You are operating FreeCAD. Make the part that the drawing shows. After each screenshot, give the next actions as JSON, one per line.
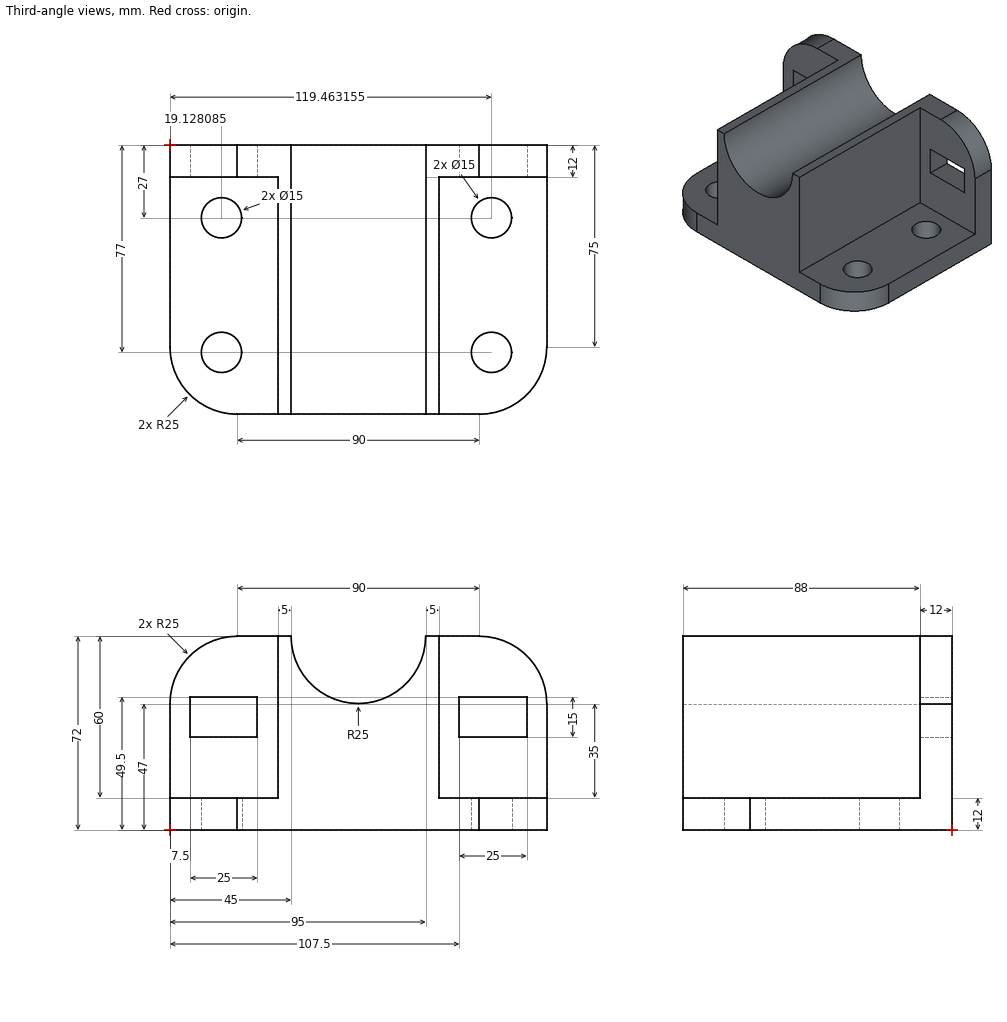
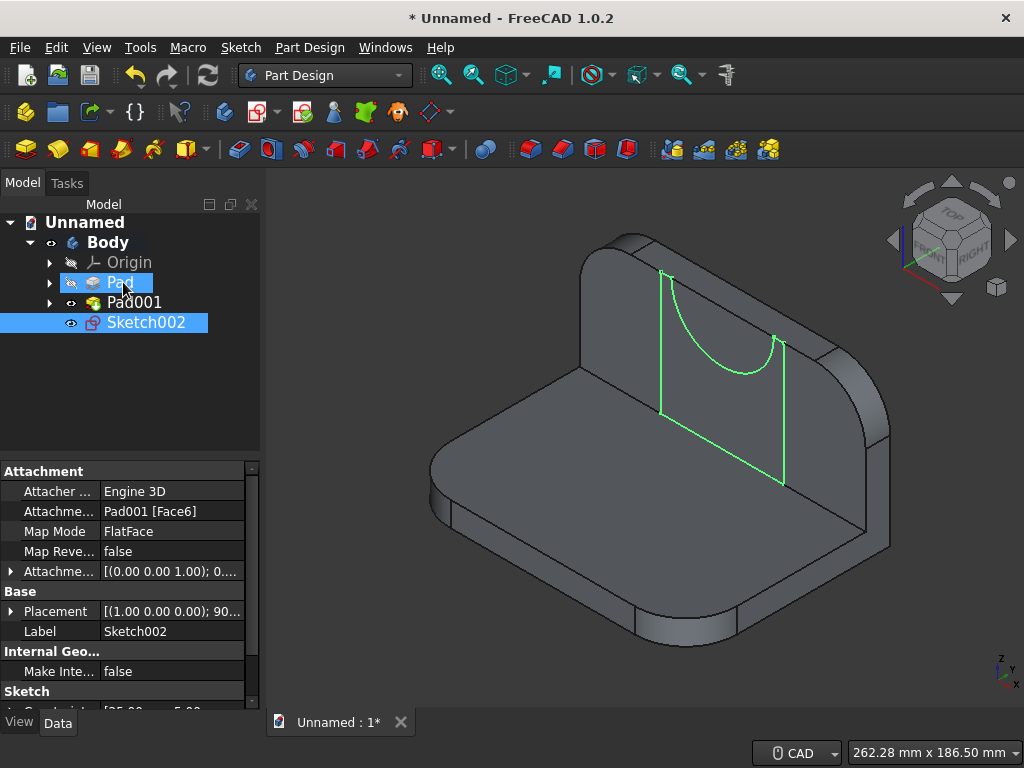
{"action": "left_click", "coordinate": [26, 150]}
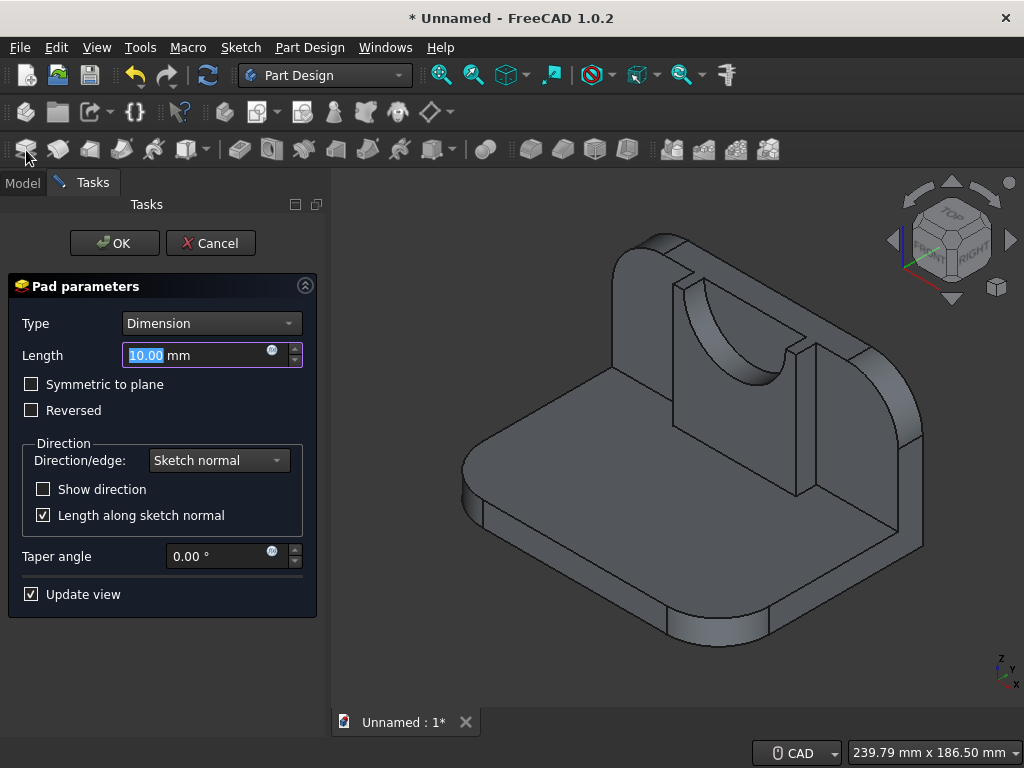
{"action": "type", "text": "88"}
{"action": "key", "text": "Tab"}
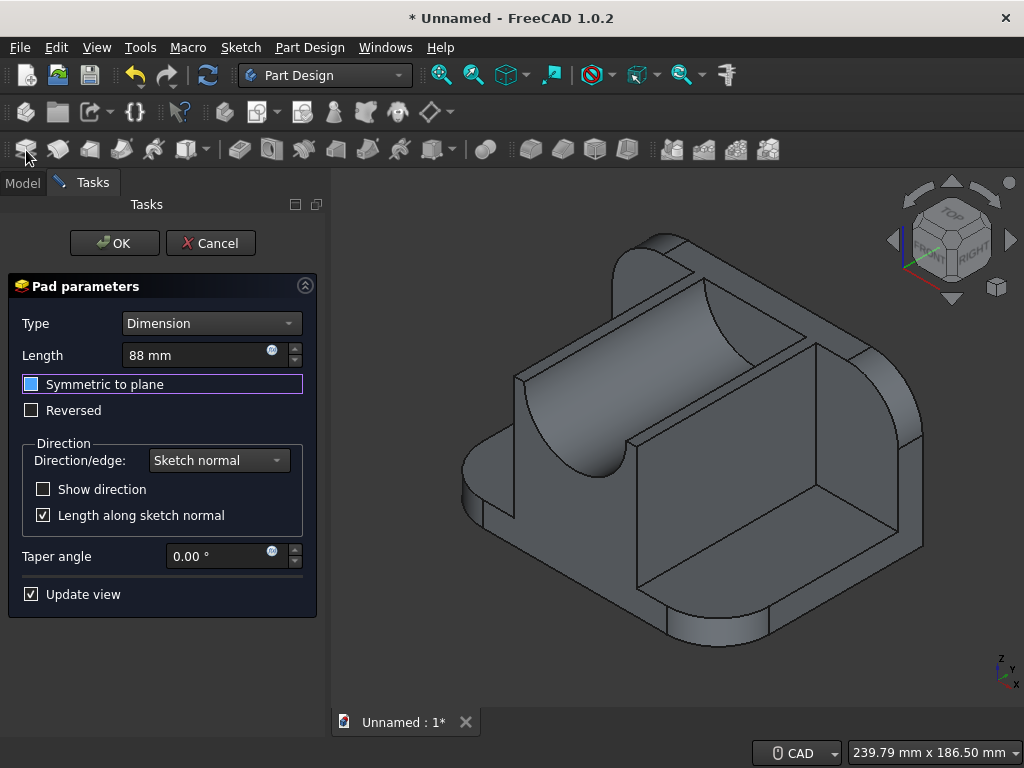
{"action": "left_click", "coordinate": [115, 243]}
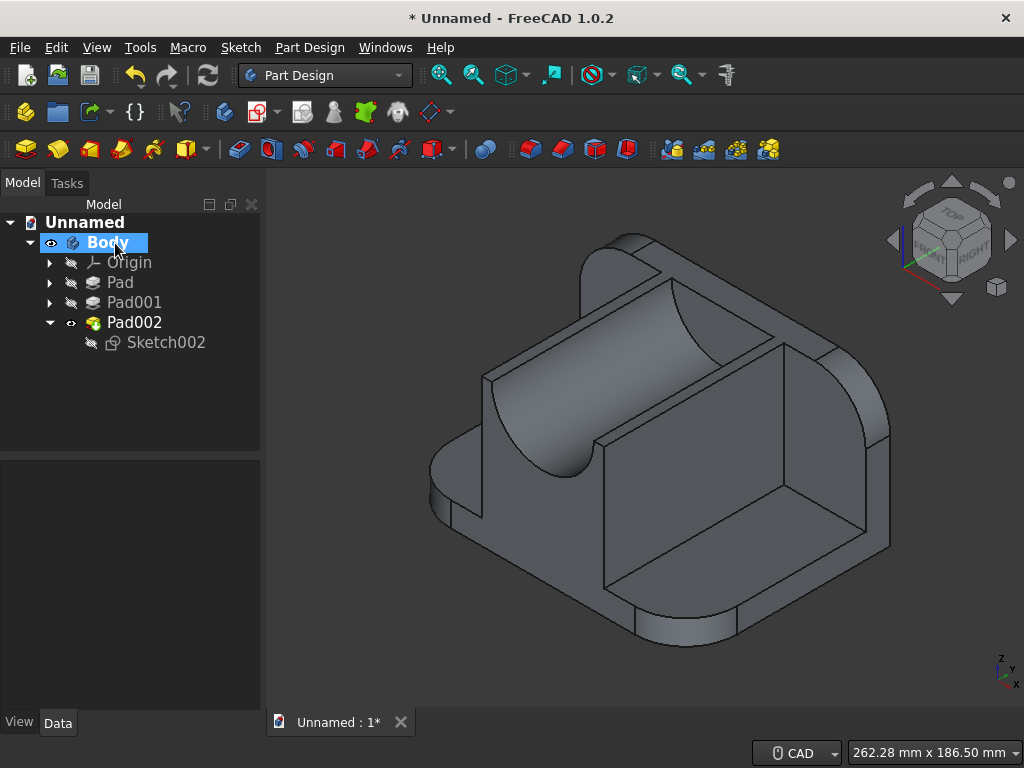
{"action": "left_click", "coordinate": [258, 112]}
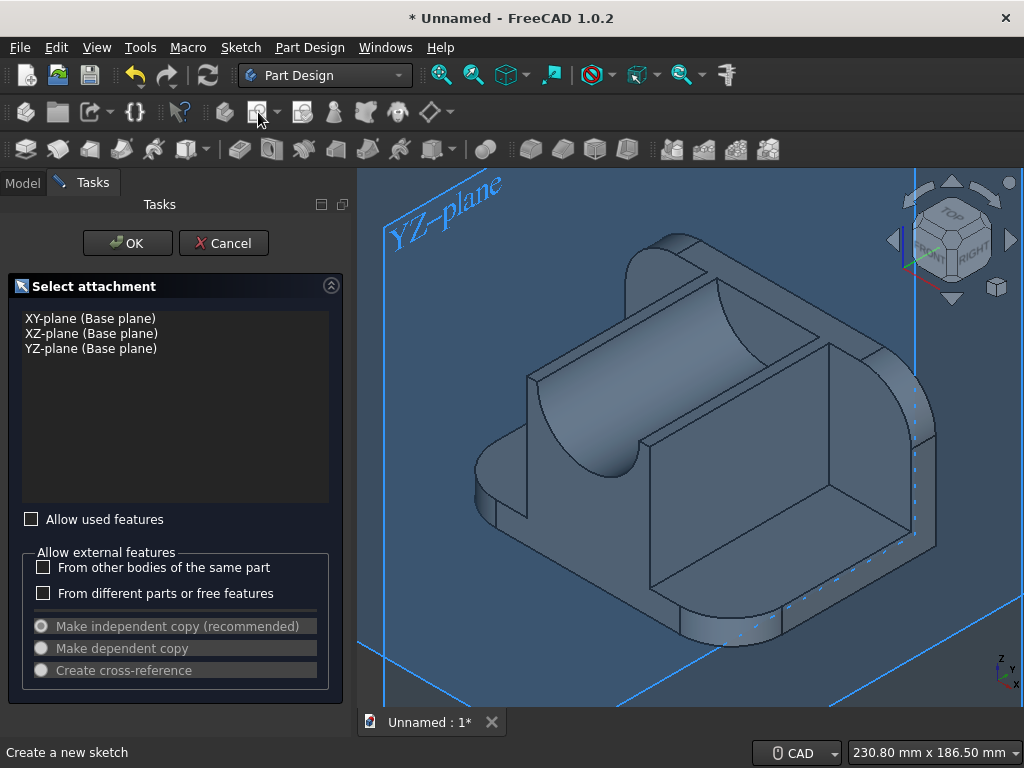
{"action": "left_click", "coordinate": [82, 334]}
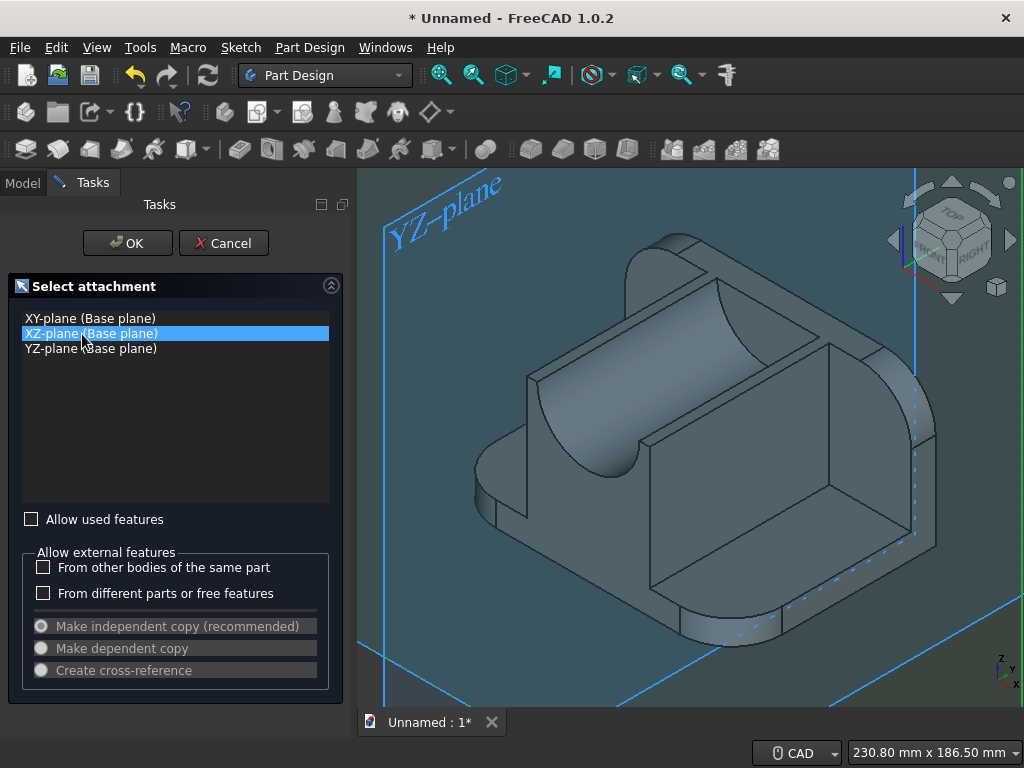
{"action": "left_click", "coordinate": [128, 243]}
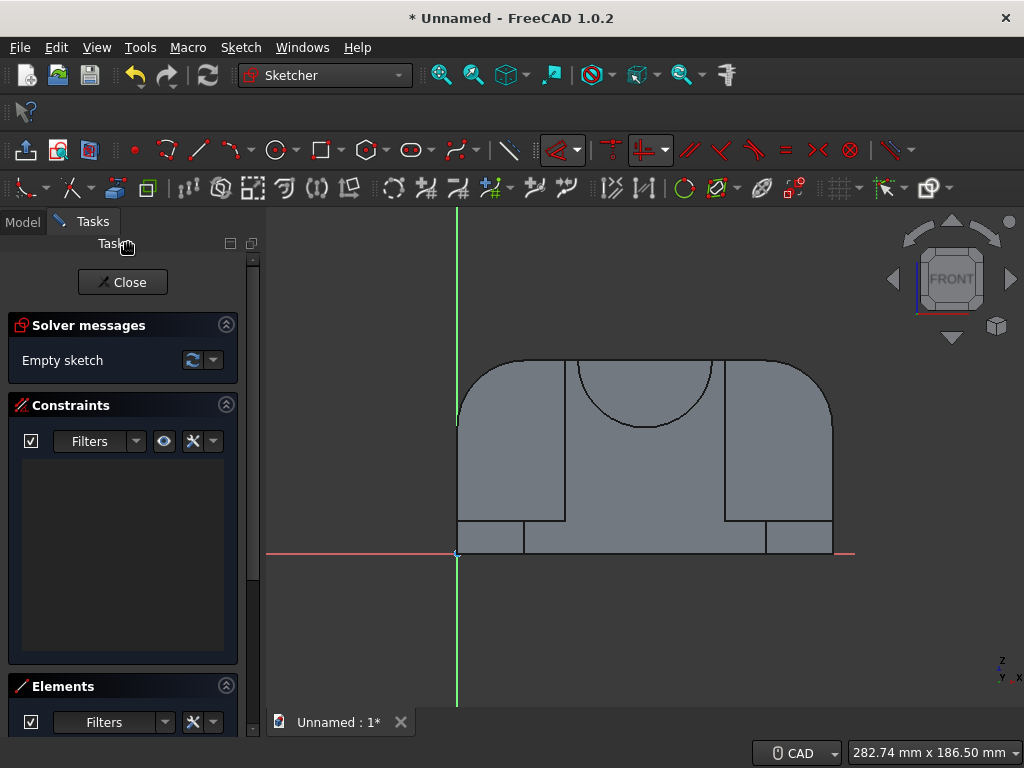
{"action": "left_click", "coordinate": [90, 150]}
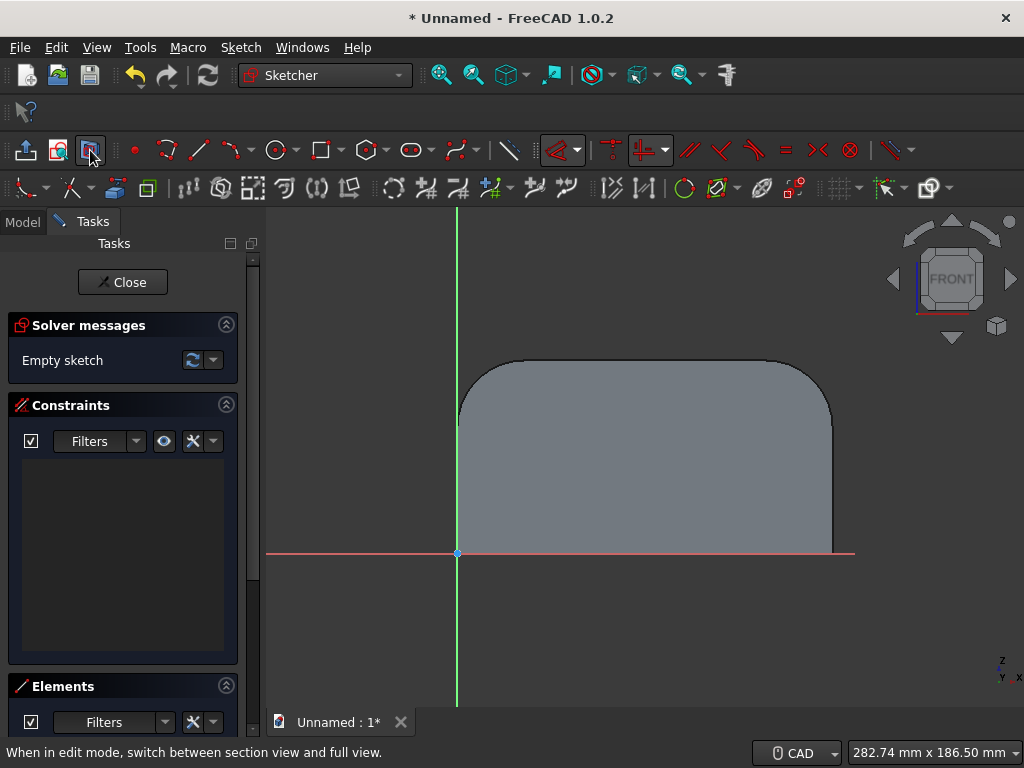
{"action": "scroll", "coordinate": [601, 457], "scroll_direction": "up", "scroll_amount": 2}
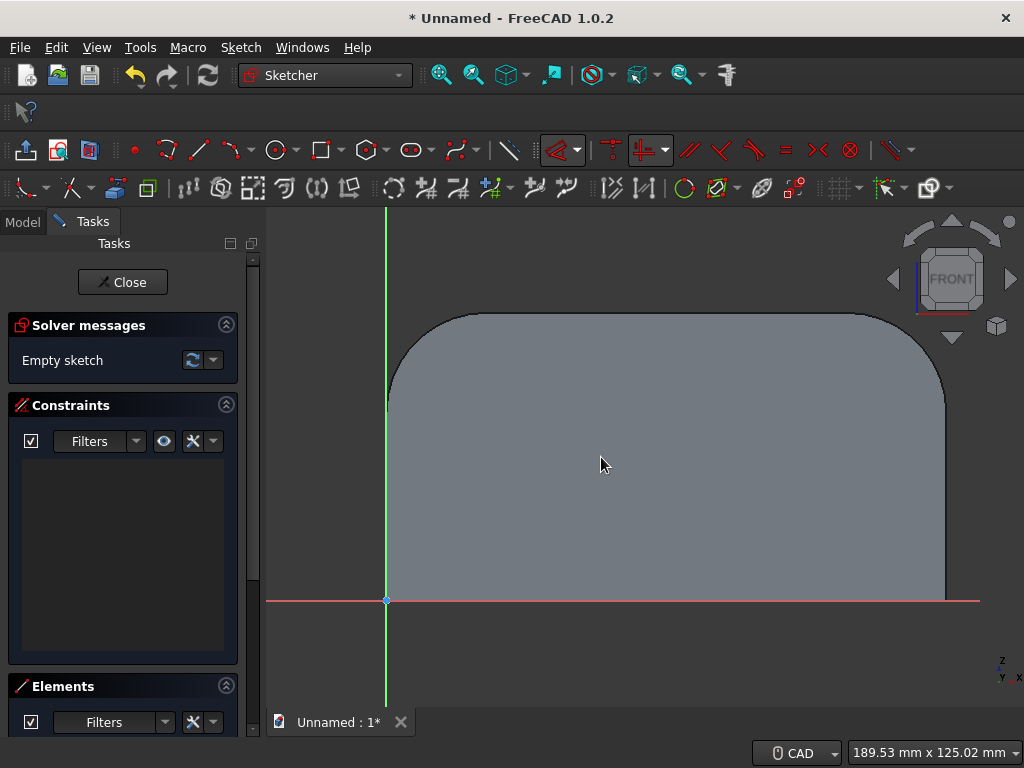
{"action": "left_click", "coordinate": [200, 150]}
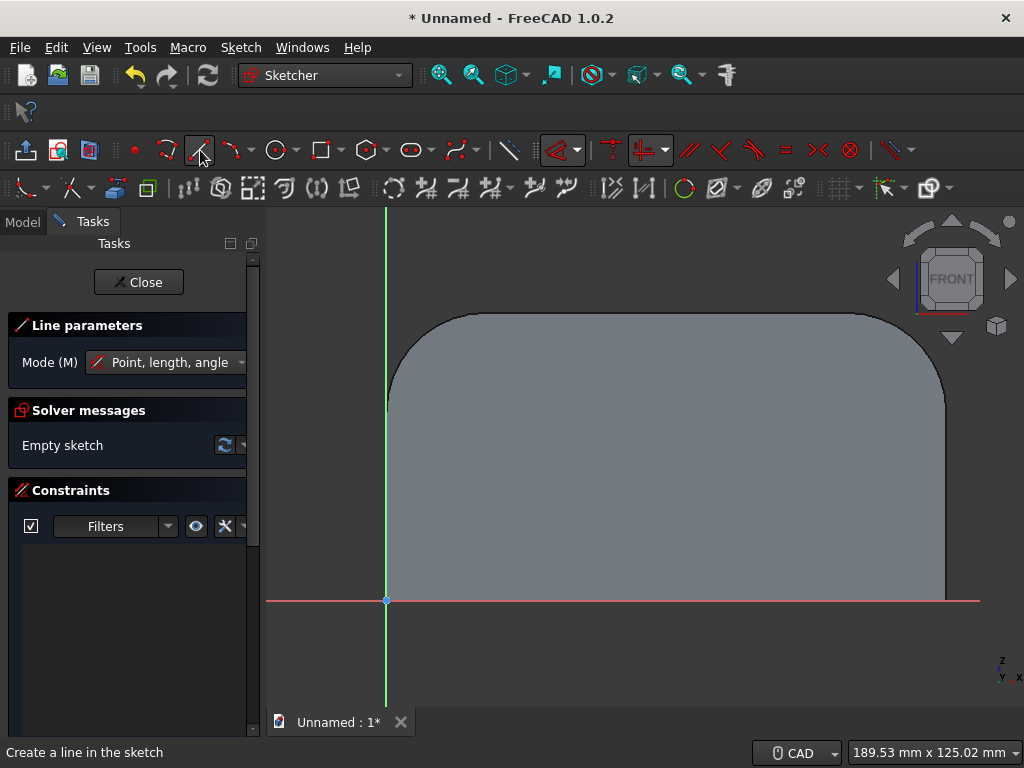
{"action": "left_click", "coordinate": [766, 313]}
{"action": "left_click", "coordinate": [566, 313]}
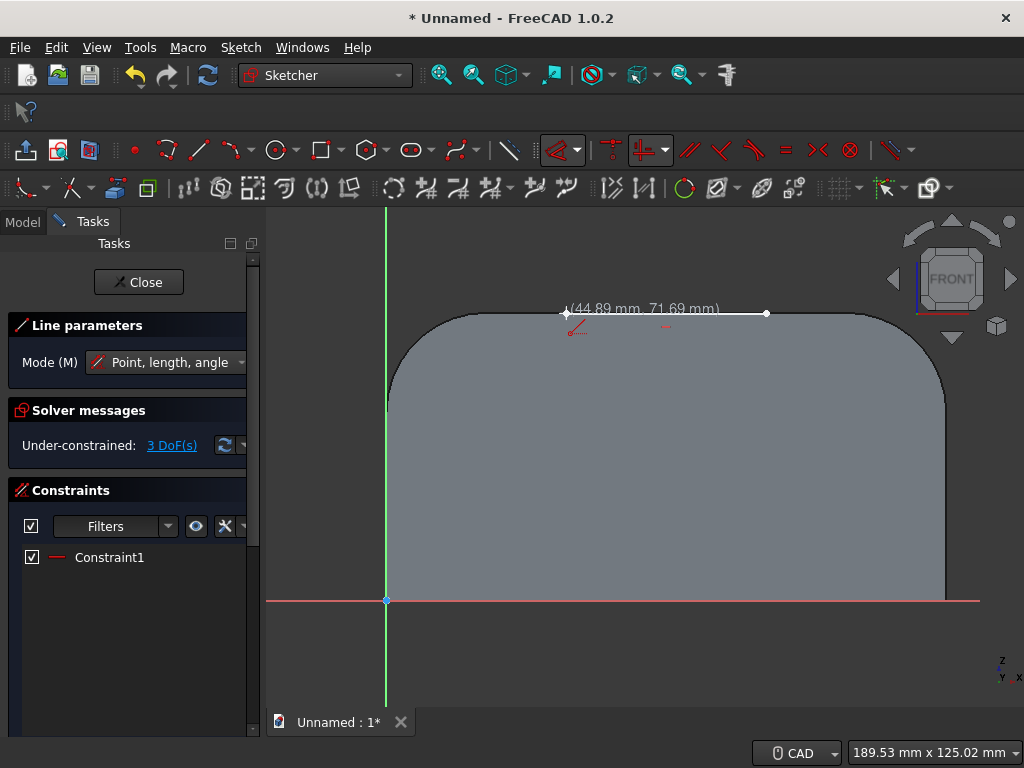
{"action": "left_click", "coordinate": [232, 150]}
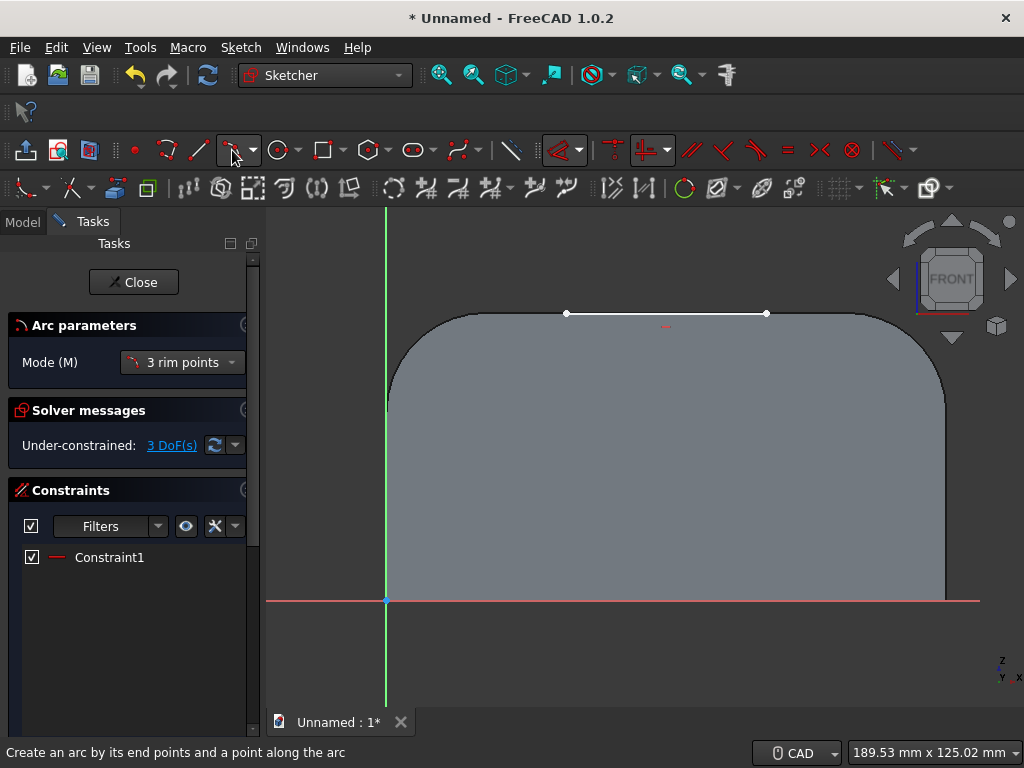
{"action": "left_click", "coordinate": [566, 314]}
{"action": "left_click", "coordinate": [766, 314]}
{"action": "left_click", "coordinate": [666, 413]}
{"action": "key", "text": "Escape"}